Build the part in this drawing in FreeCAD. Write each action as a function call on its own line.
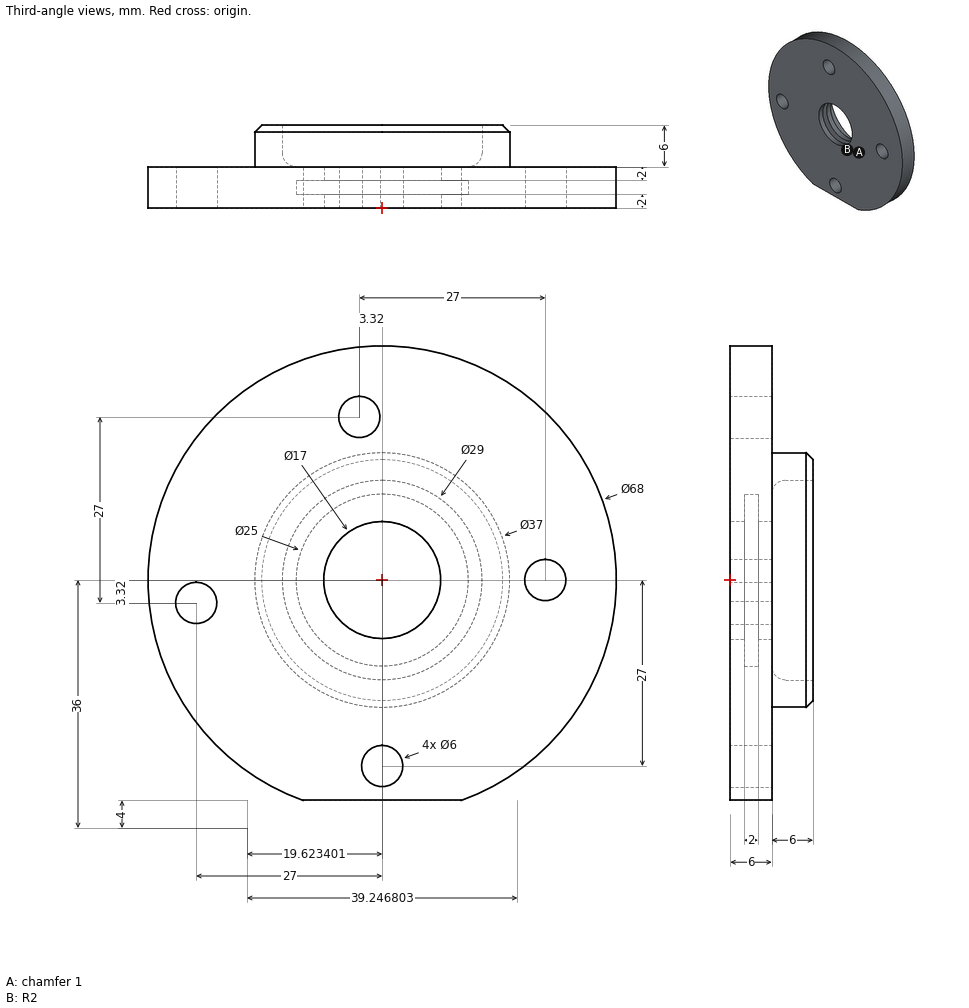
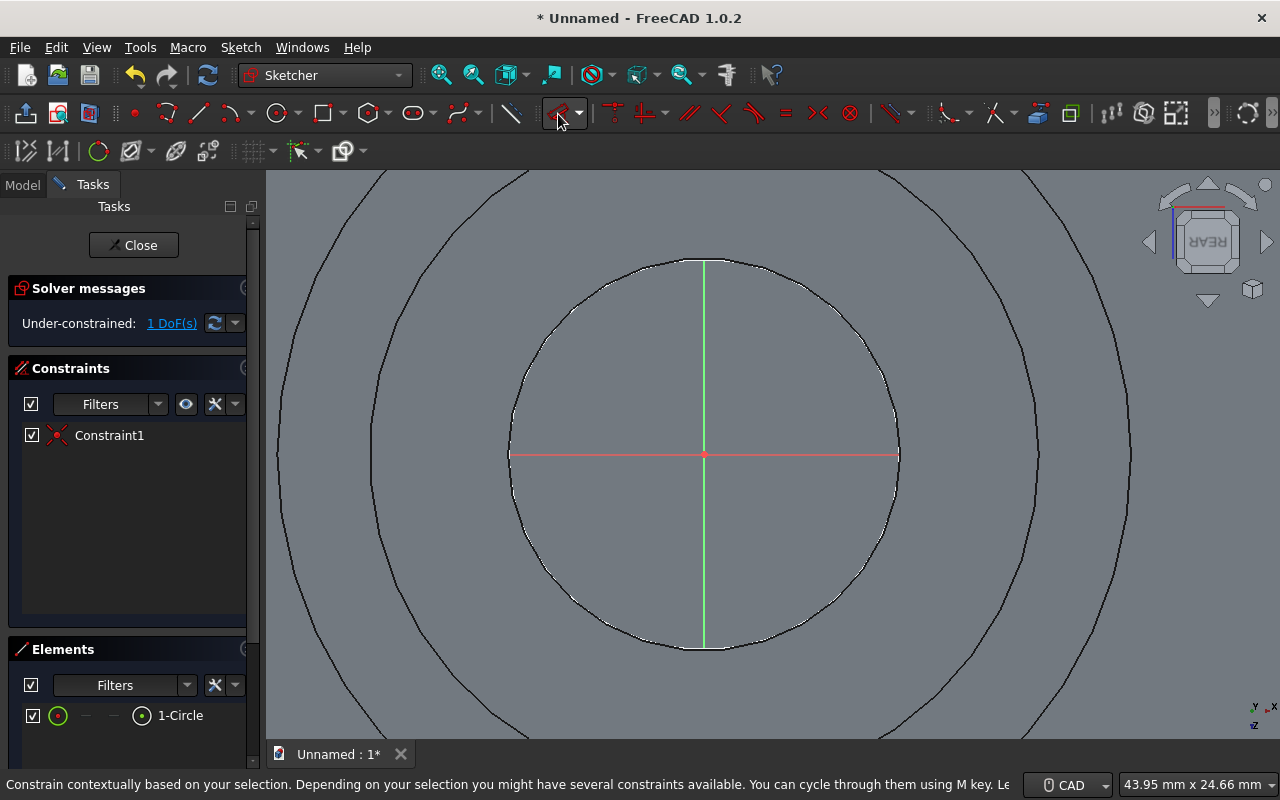
click(842, 316)
click(865, 293)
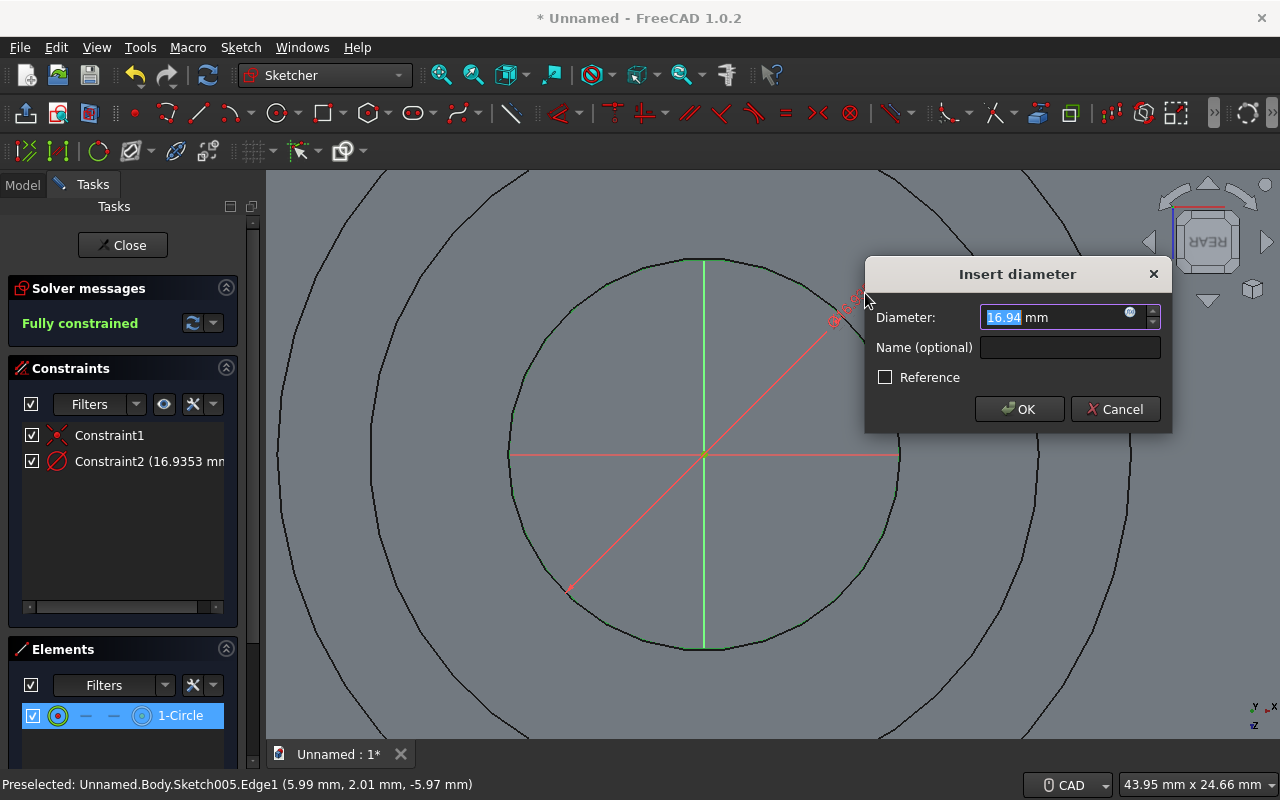
text(17)
key(Return)
key(Escape)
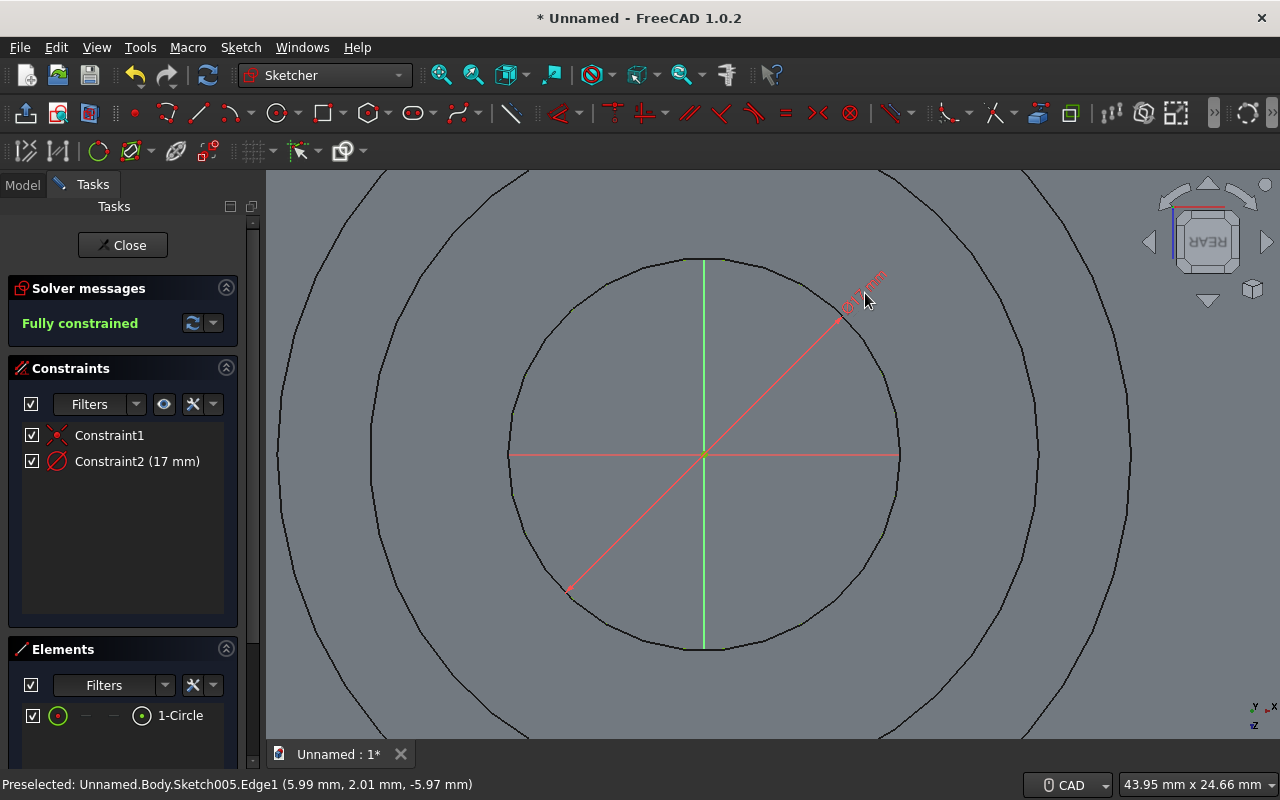
click(123, 245)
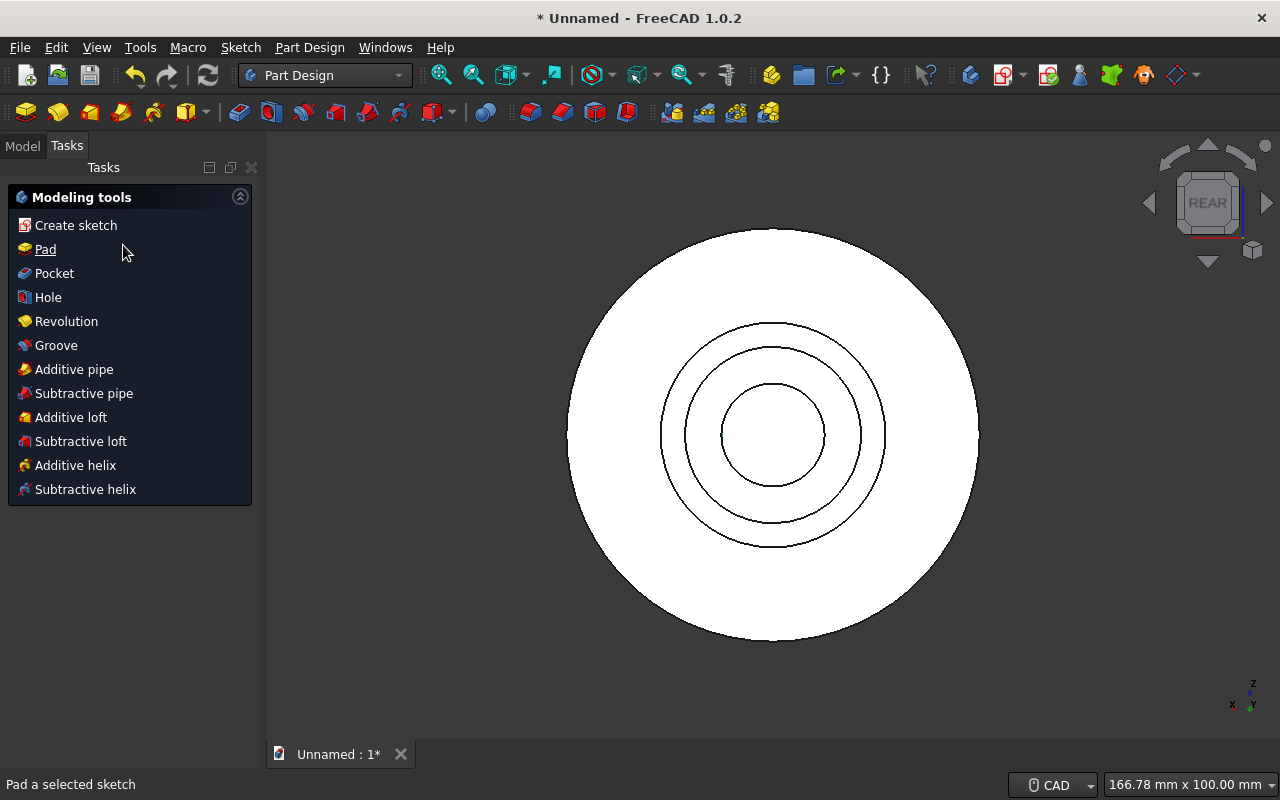
click(240, 112)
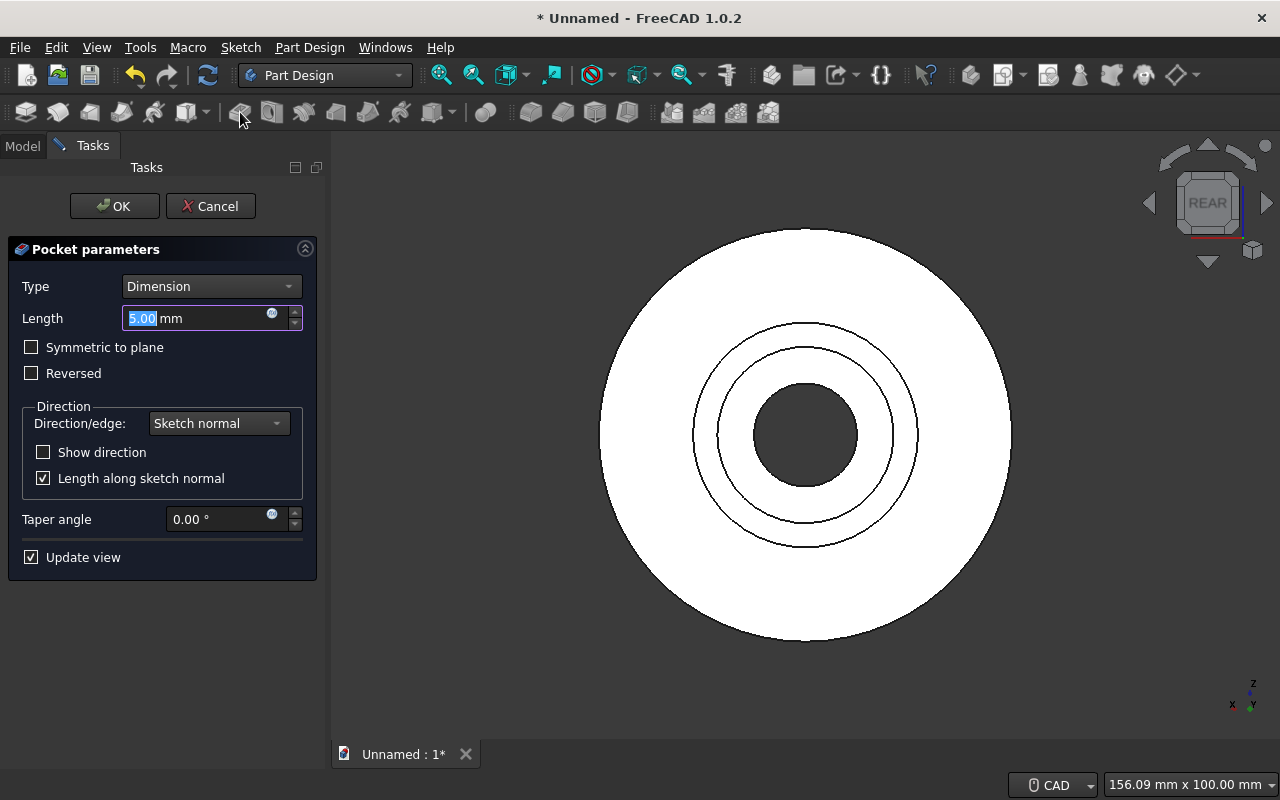
text(2)
key(Tab)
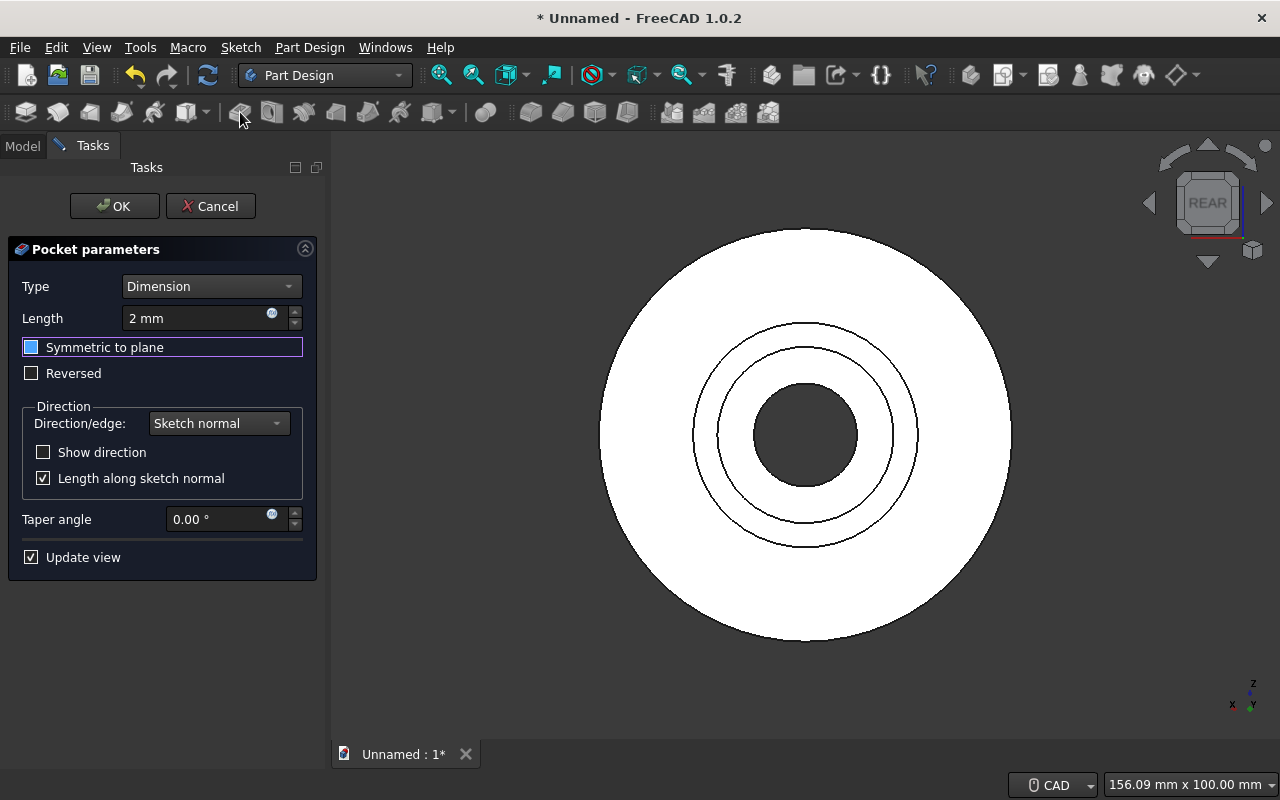
click(115, 206)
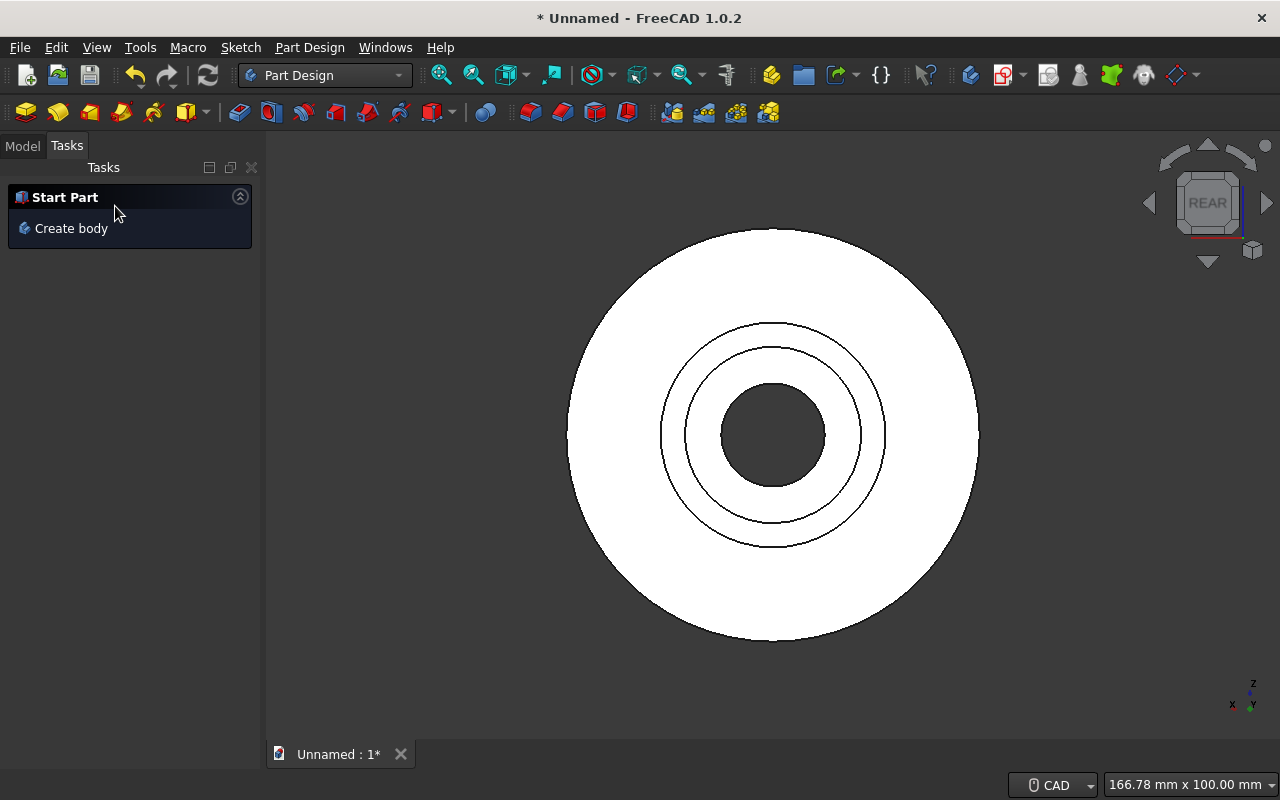
click(885, 434)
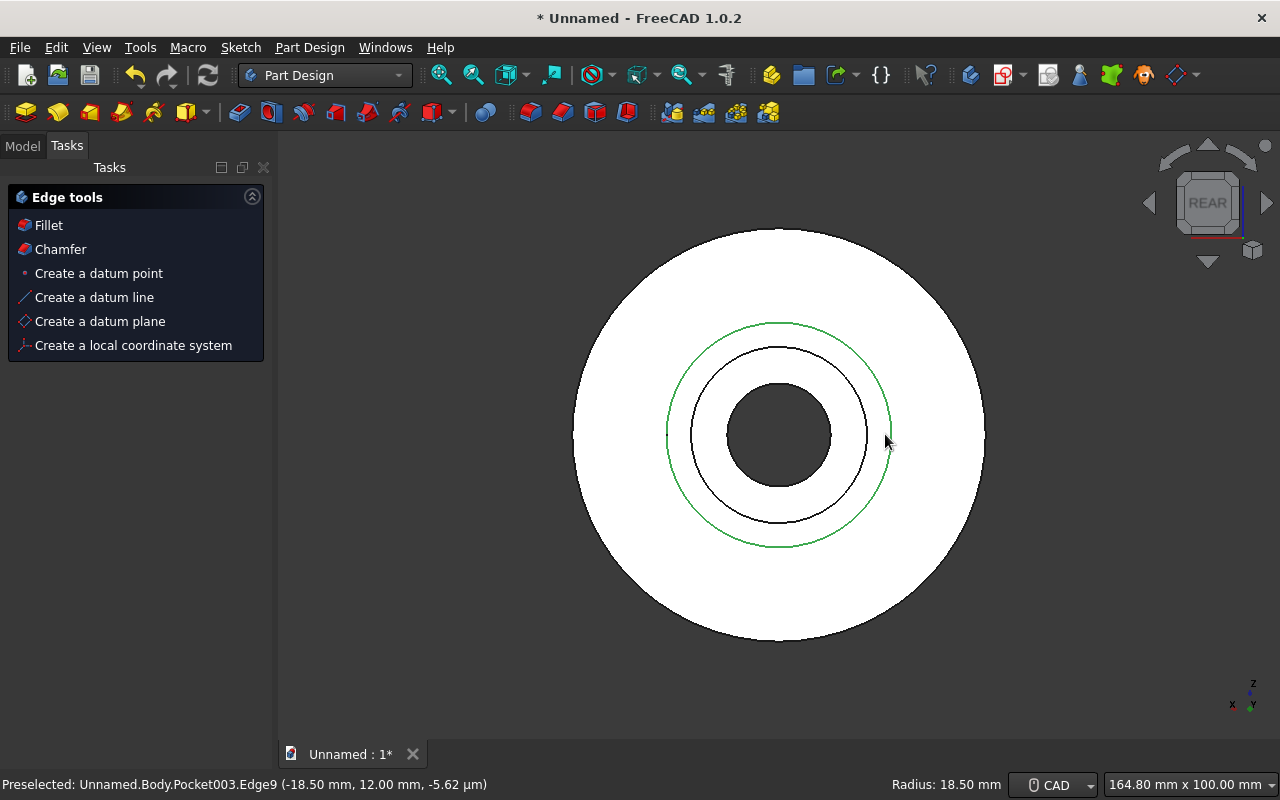
click(564, 112)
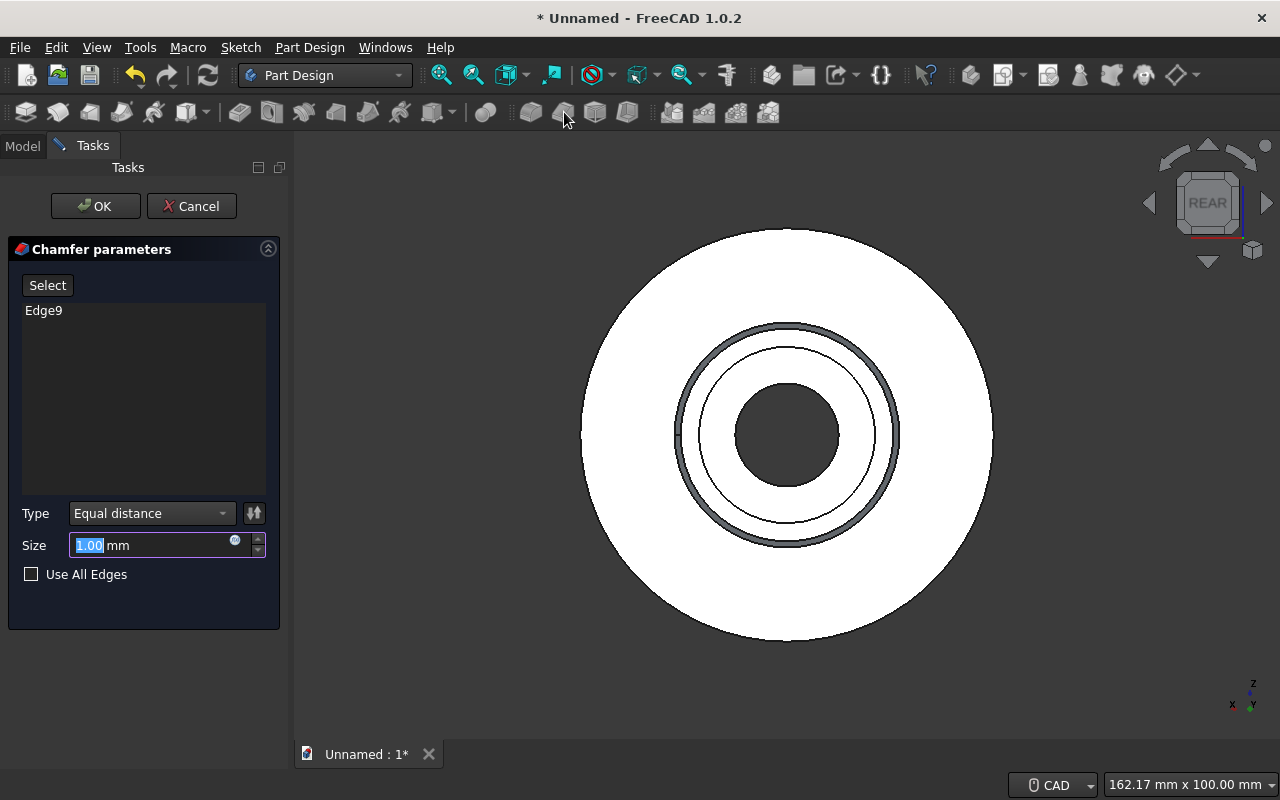
text(1)
key(Tab)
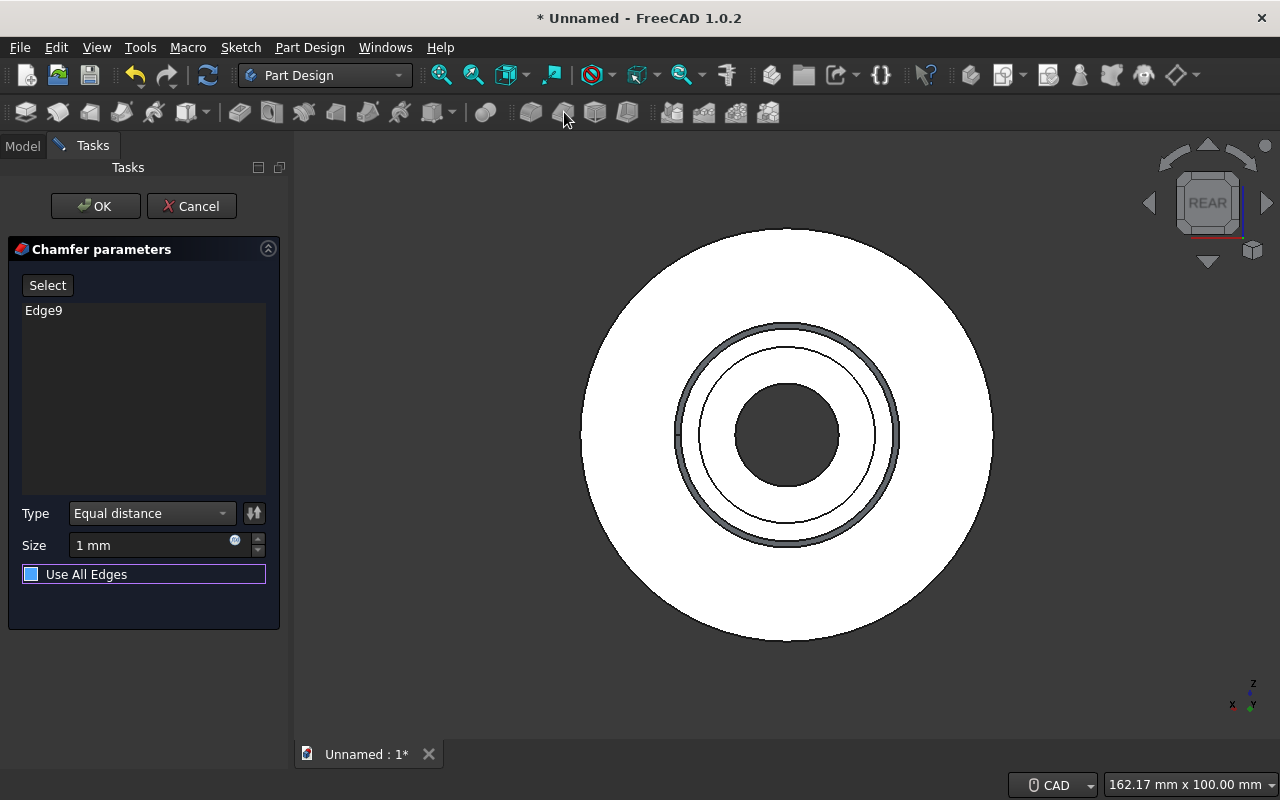
click(96, 206)